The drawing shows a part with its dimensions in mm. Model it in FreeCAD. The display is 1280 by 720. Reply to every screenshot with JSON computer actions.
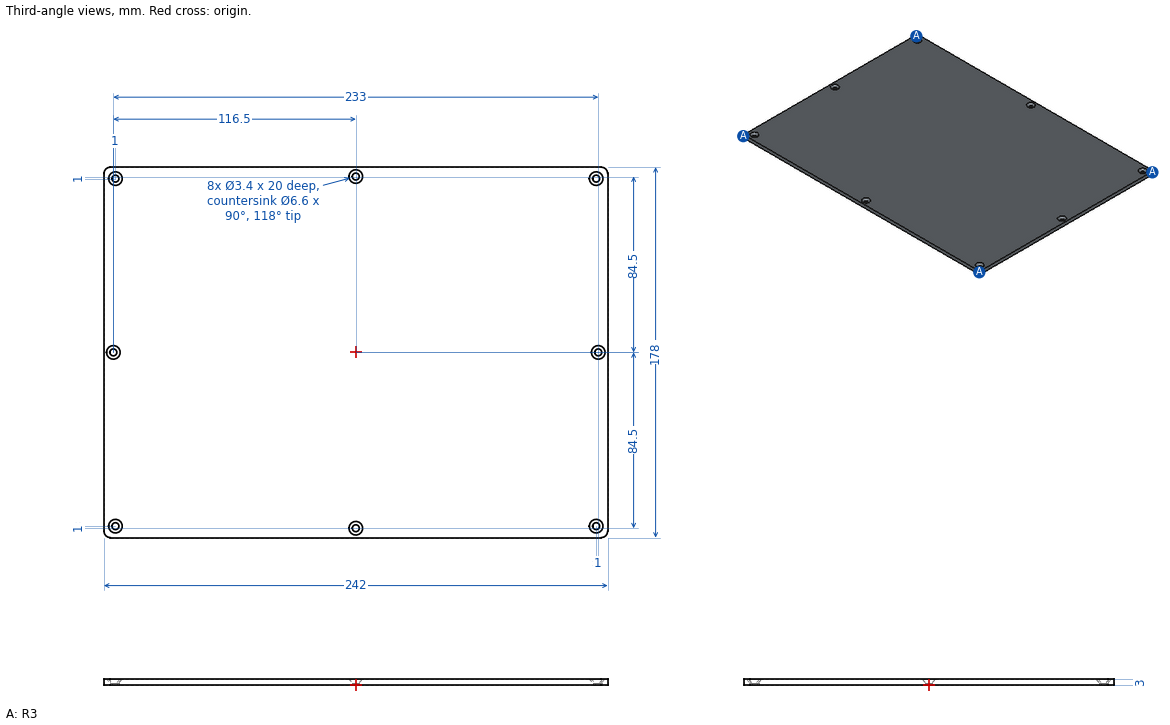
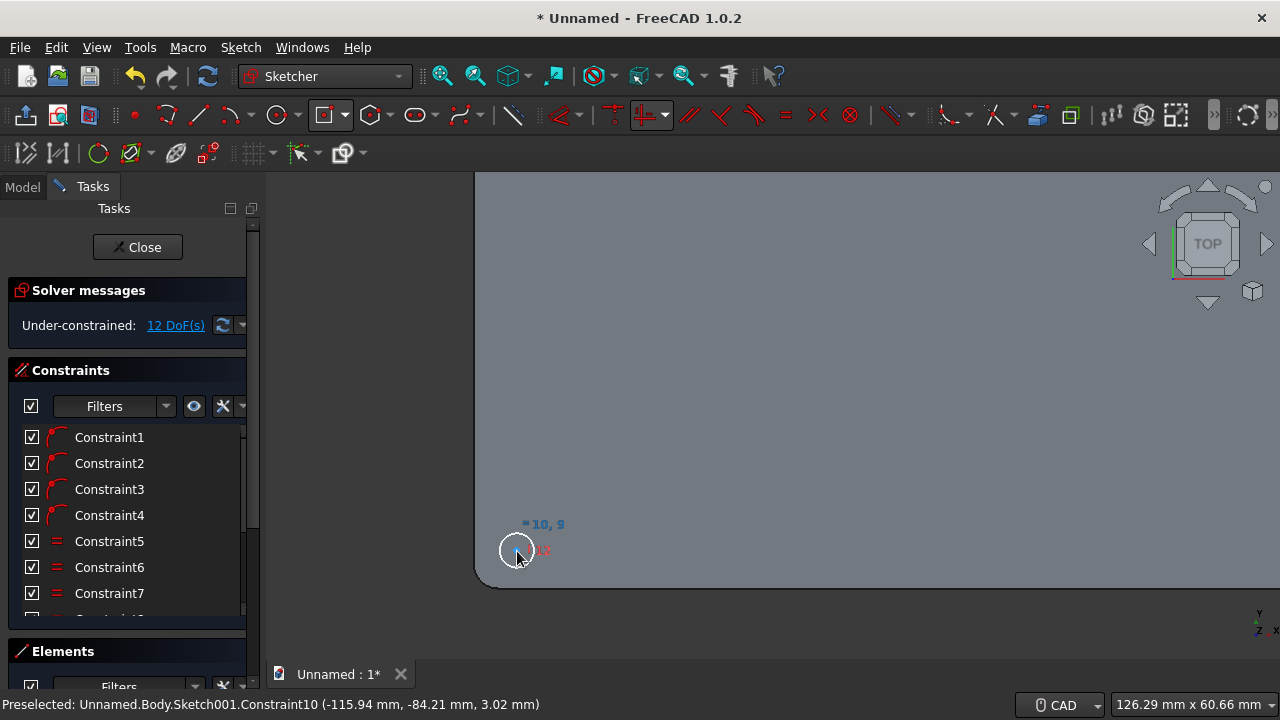
{"action": "left_click", "coordinate": [517, 550]}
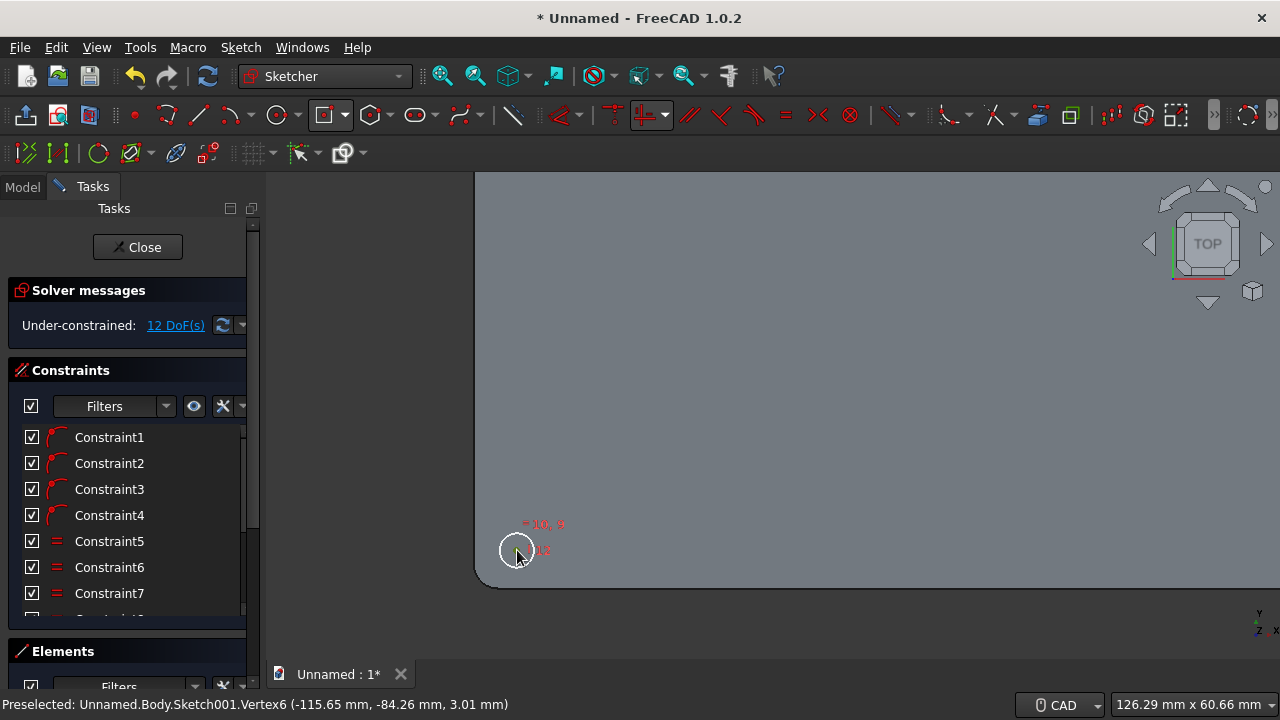
{"action": "scroll", "coordinate": [517, 552], "scroll_direction": "down", "scroll_amount": 8}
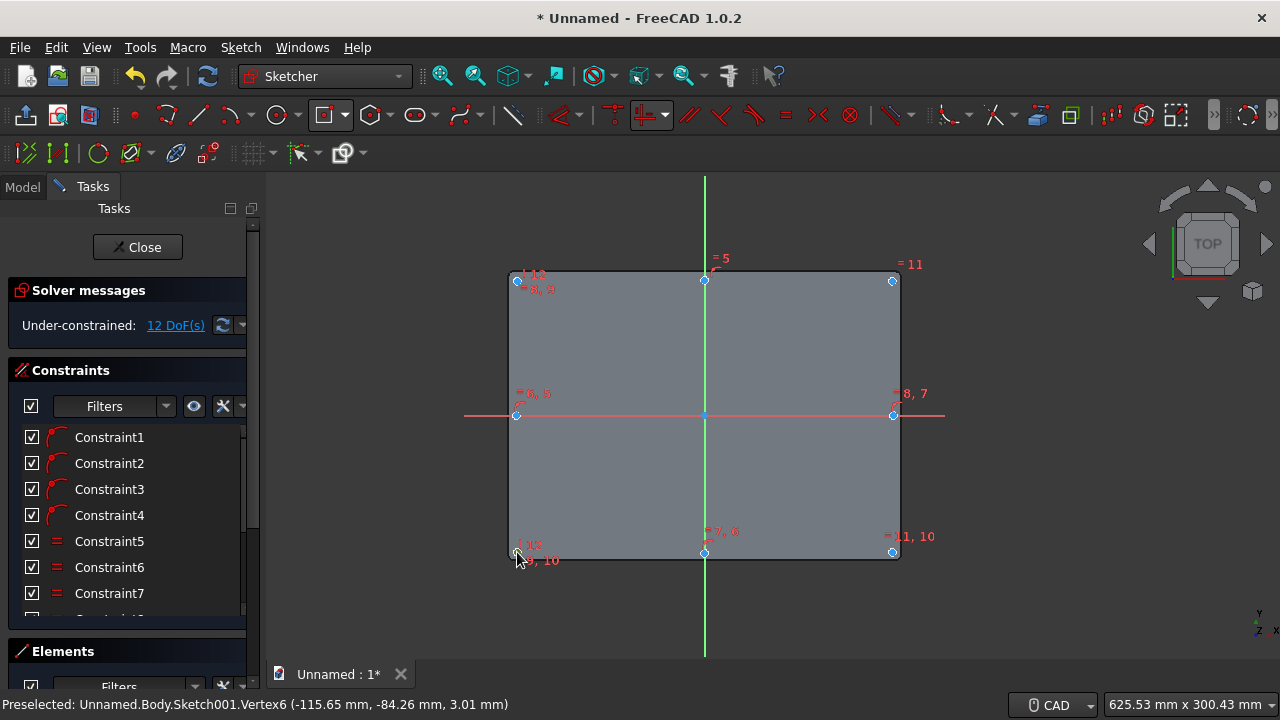
{"action": "left_click", "coordinate": [892, 552]}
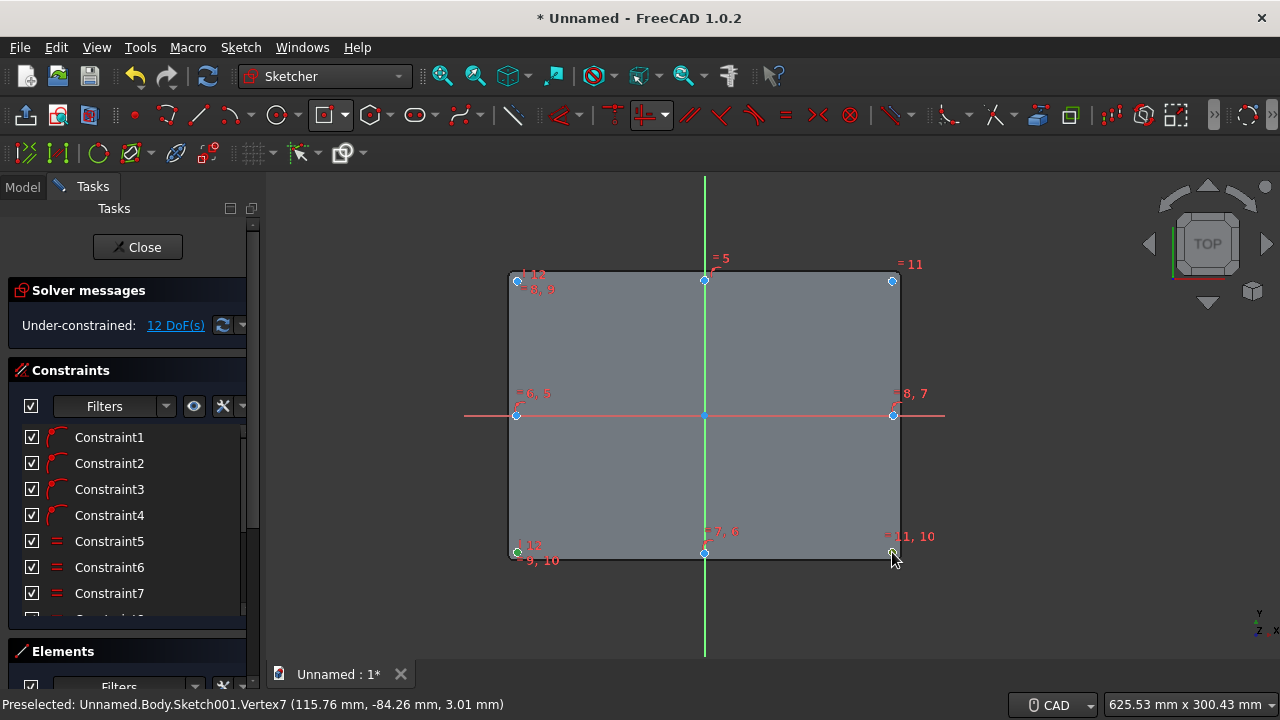
{"action": "key", "text": "h"}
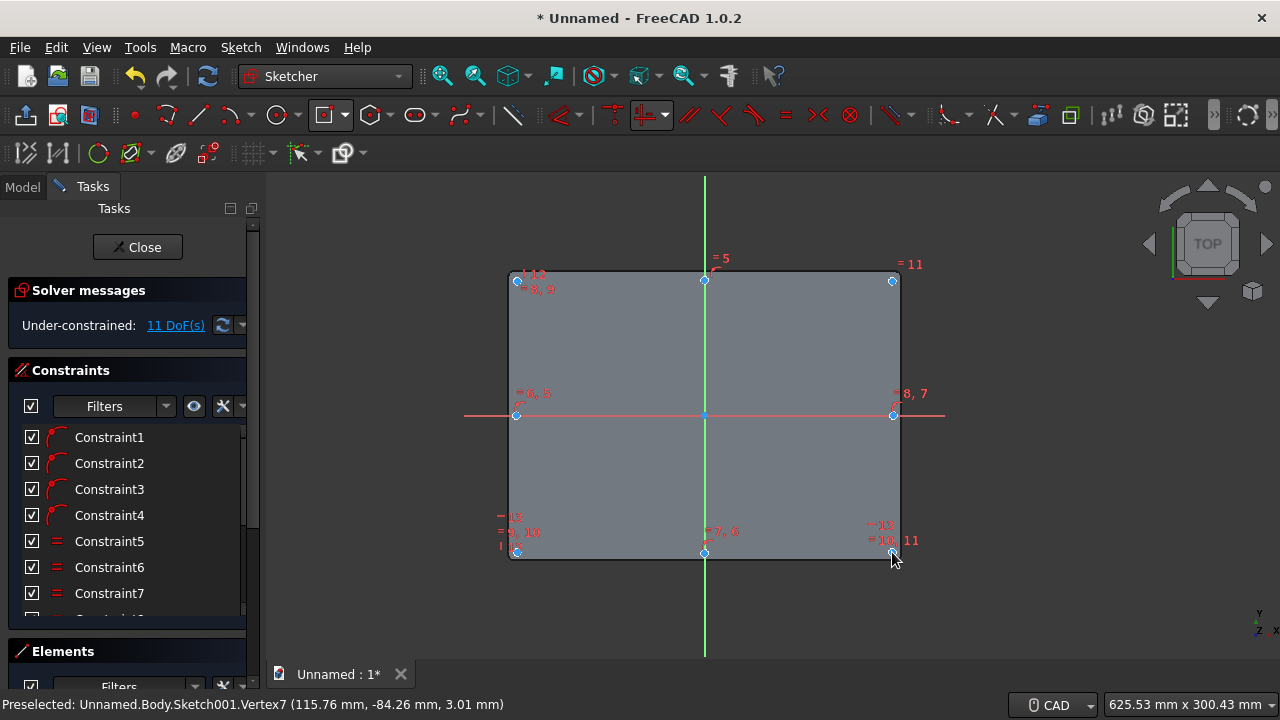
{"action": "left_click", "coordinate": [892, 552]}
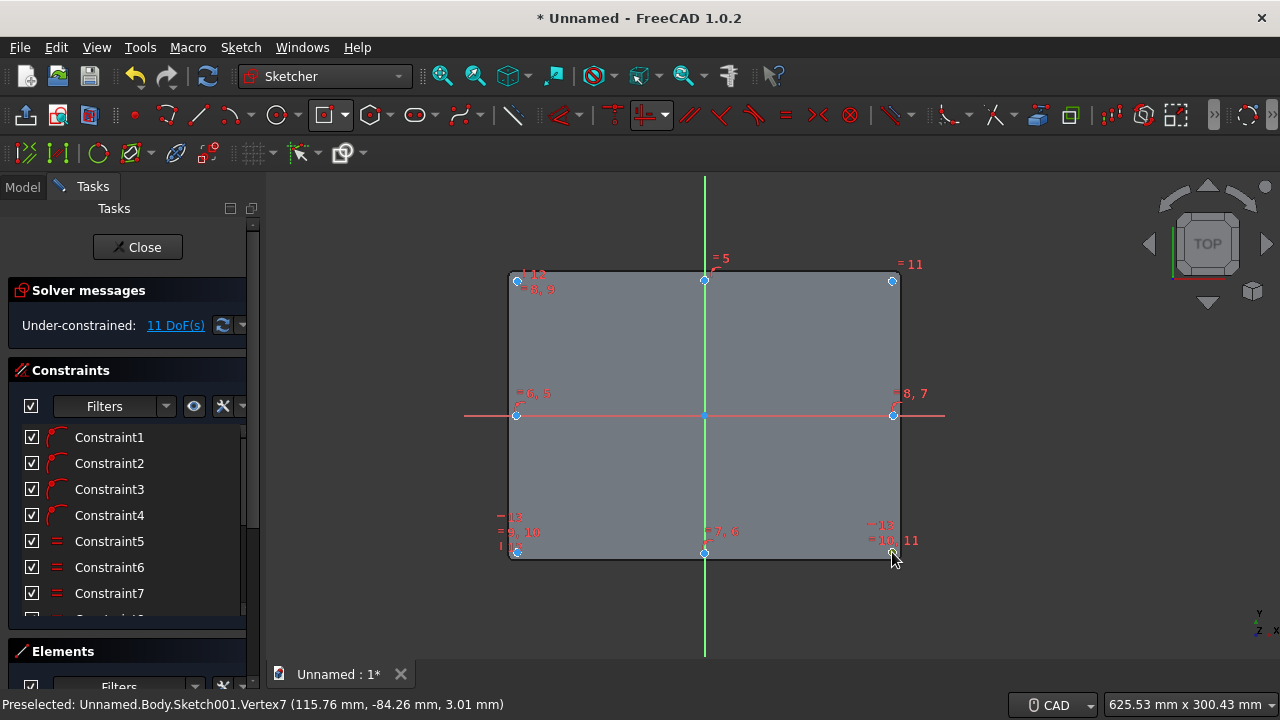
{"action": "left_click", "coordinate": [892, 281]}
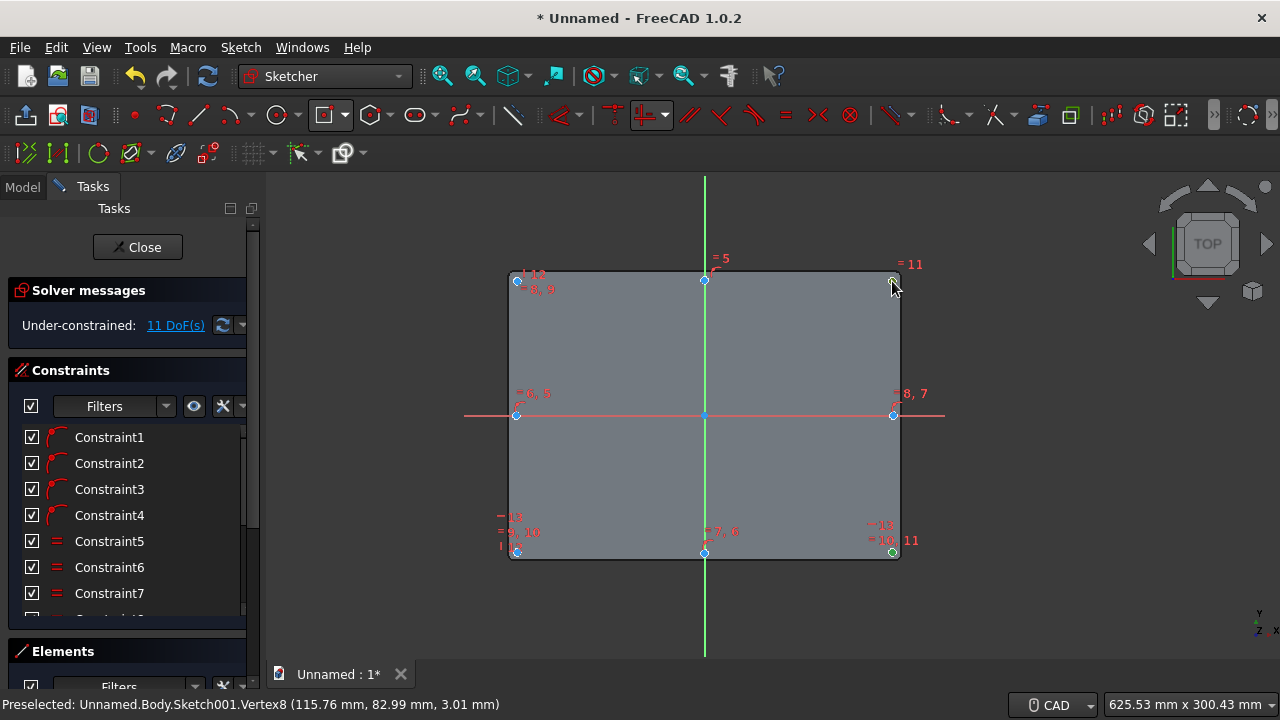
{"action": "left_click", "coordinate": [668, 116]}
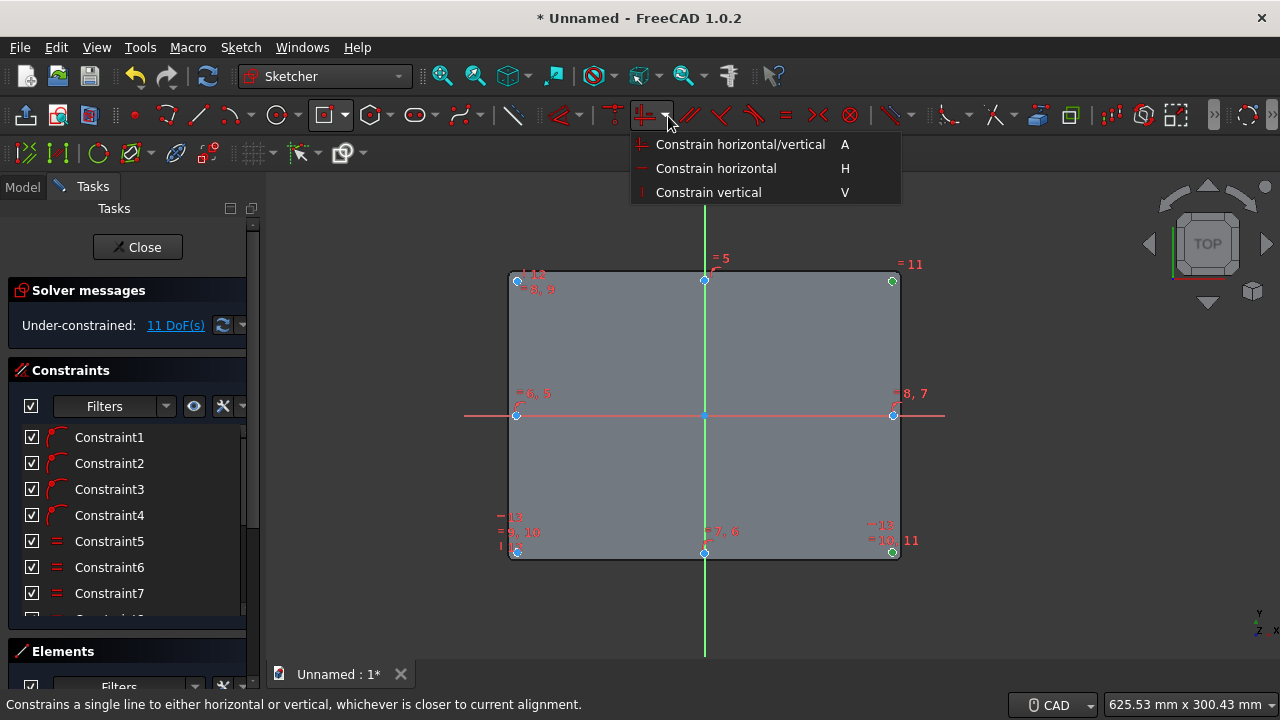
{"action": "left_click", "coordinate": [766, 192]}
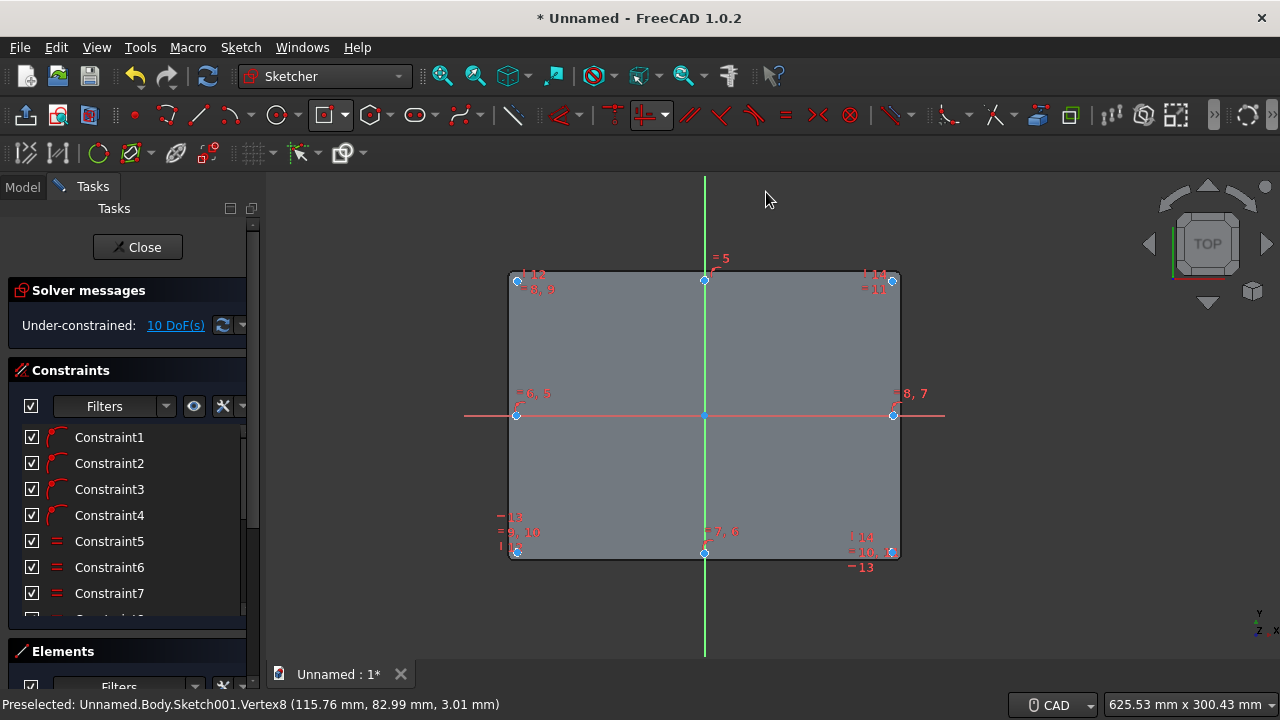
{"action": "left_click", "coordinate": [517, 281]}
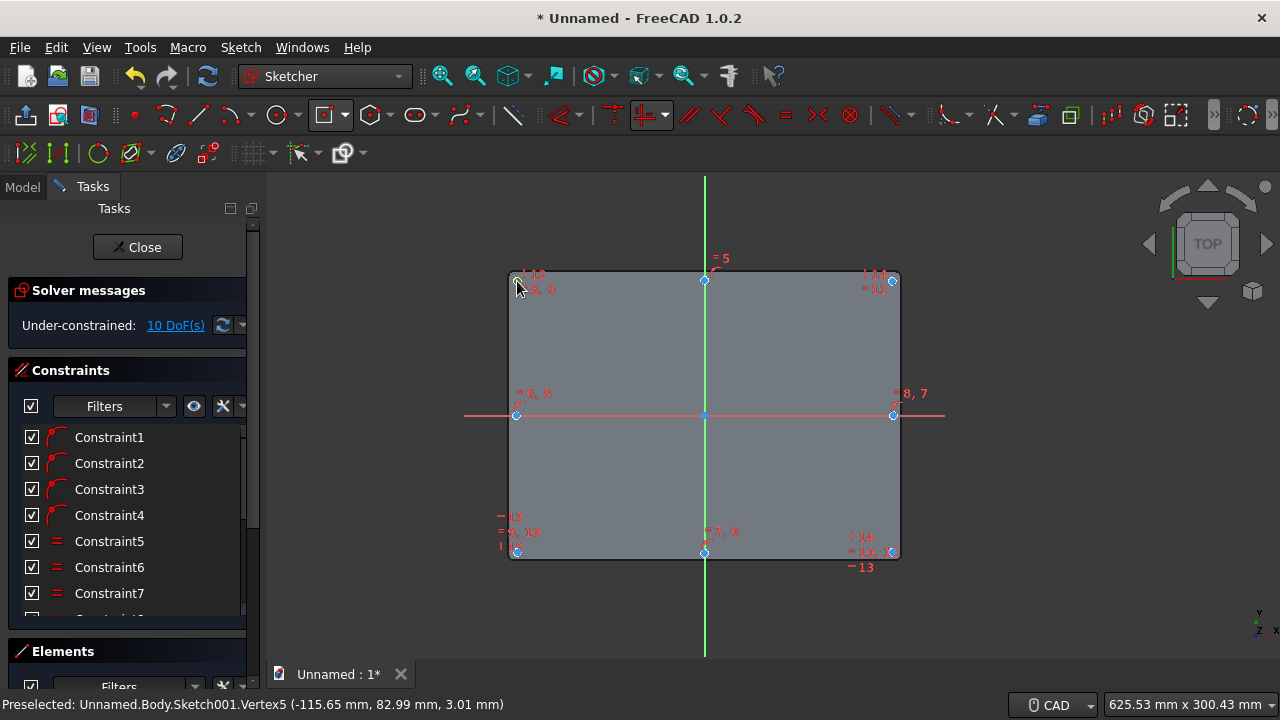
{"action": "left_click", "coordinate": [892, 281]}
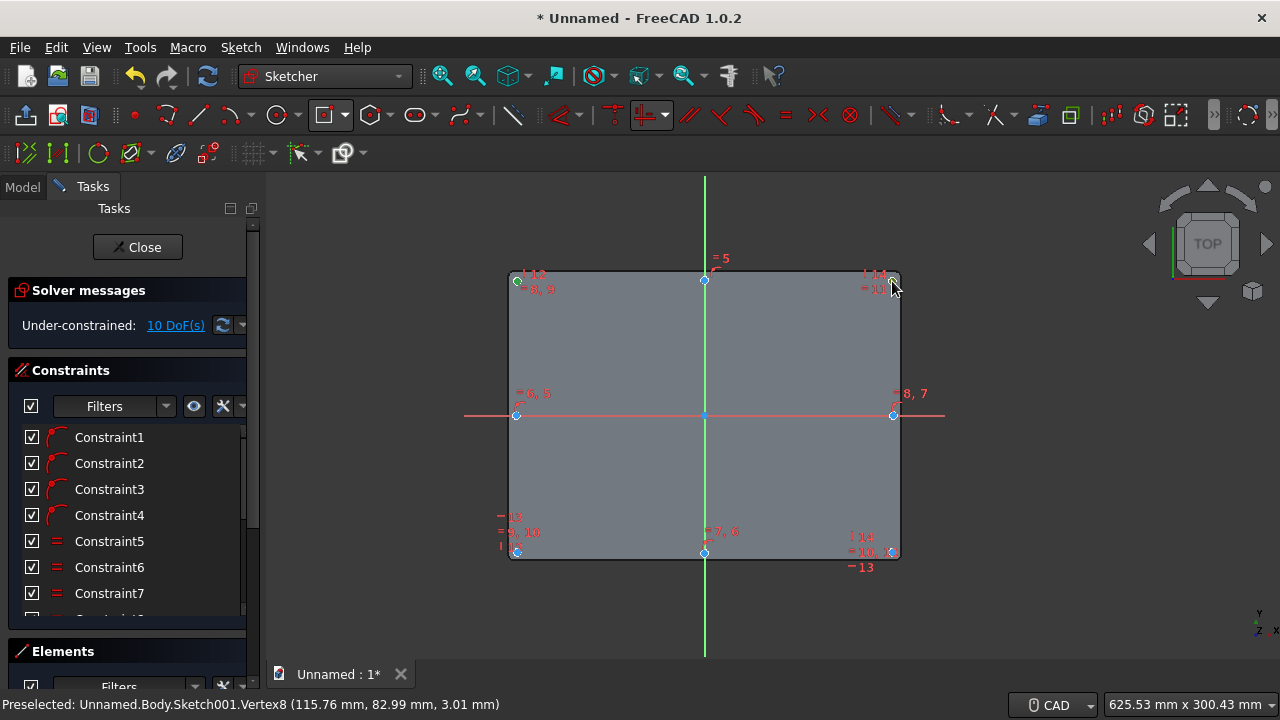
{"action": "left_click", "coordinate": [668, 116]}